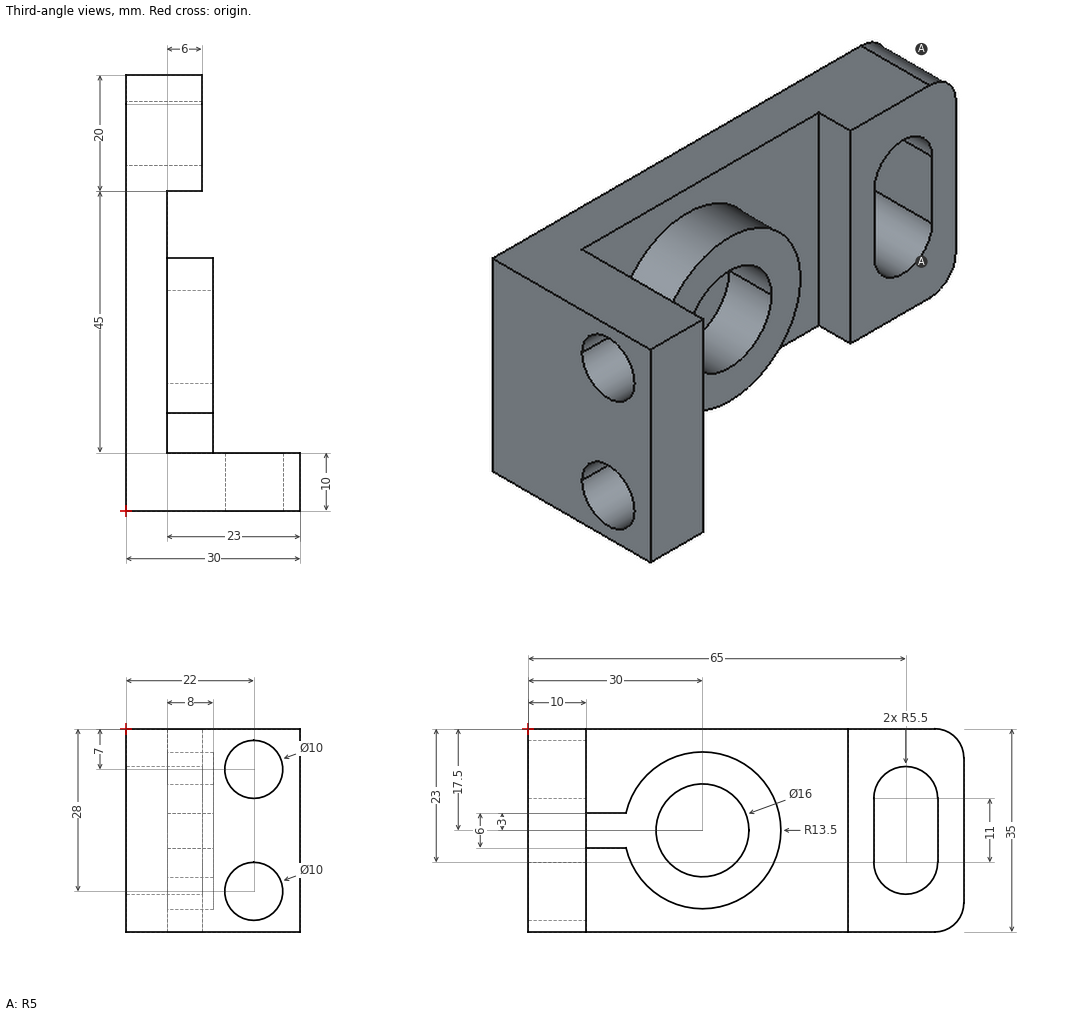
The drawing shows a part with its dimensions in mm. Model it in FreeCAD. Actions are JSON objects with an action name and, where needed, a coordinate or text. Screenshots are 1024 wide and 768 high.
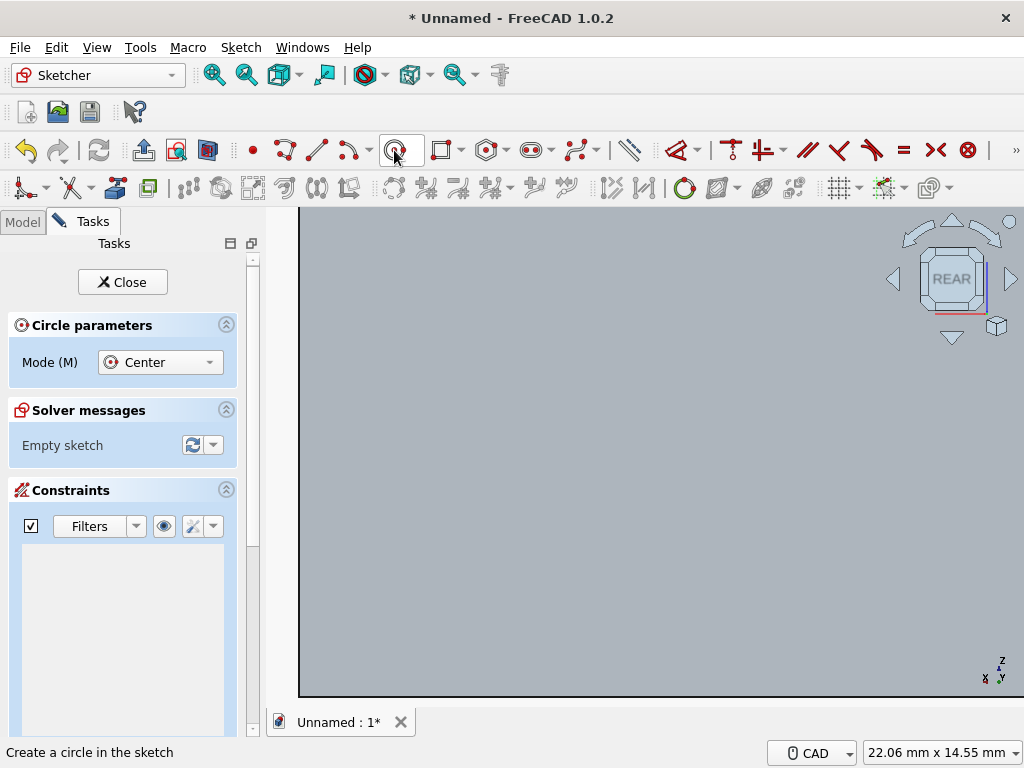
{"action": "left_click", "coordinate": [574, 456]}
{"action": "left_click", "coordinate": [695, 335]}
{"action": "key", "text": "Escape"}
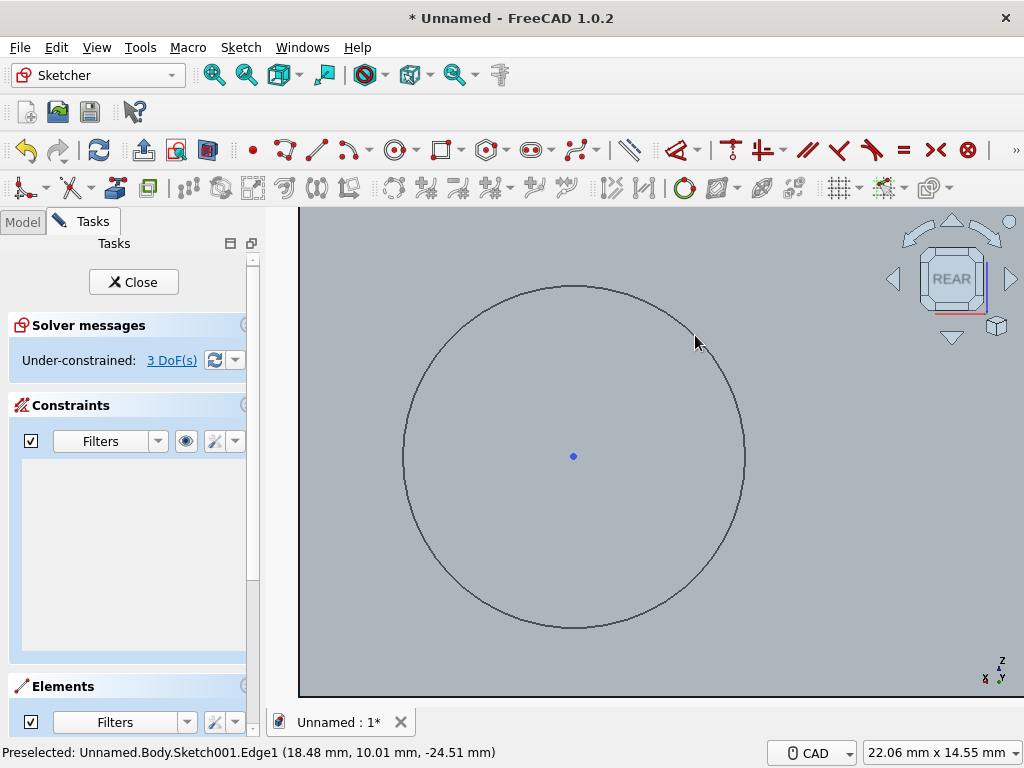
{"action": "left_click", "coordinate": [676, 150]}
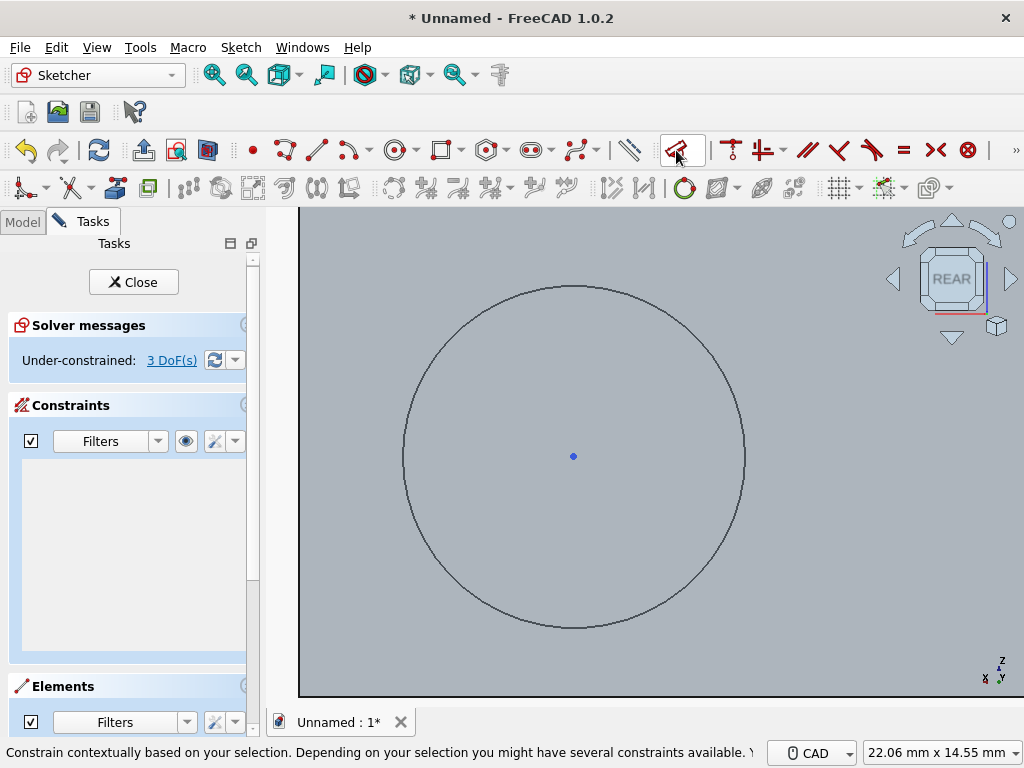
{"action": "left_click", "coordinate": [695, 336]}
{"action": "left_click", "coordinate": [718, 313]}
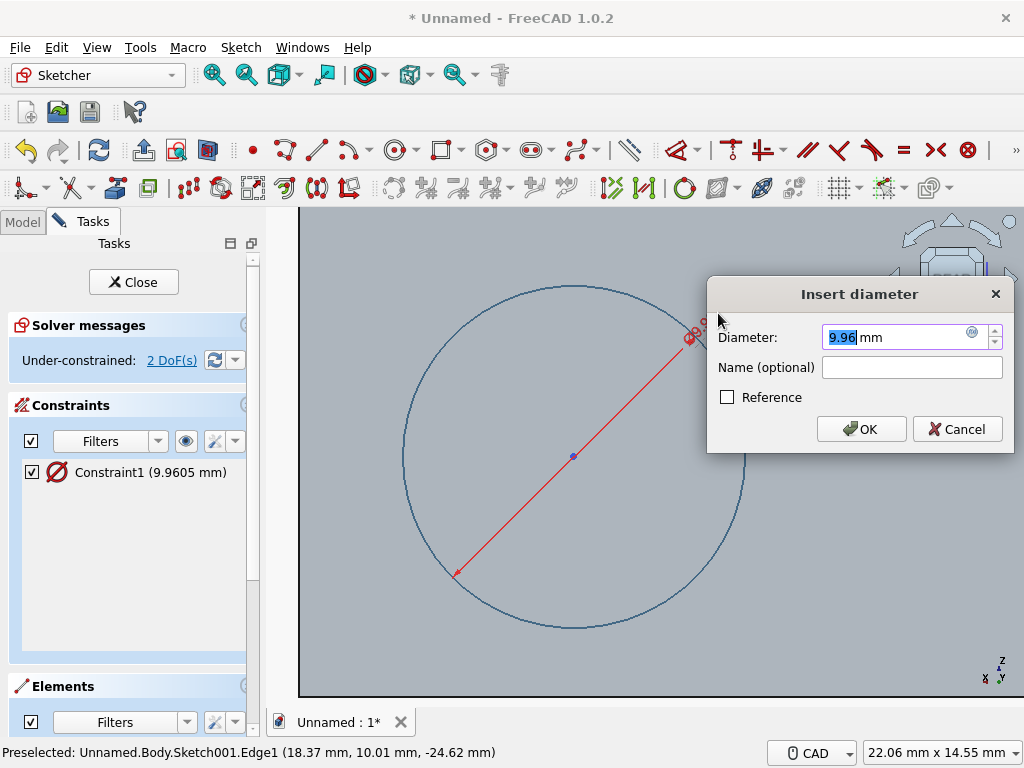
{"action": "type", "text": "10"}
{"action": "key", "text": "Return"}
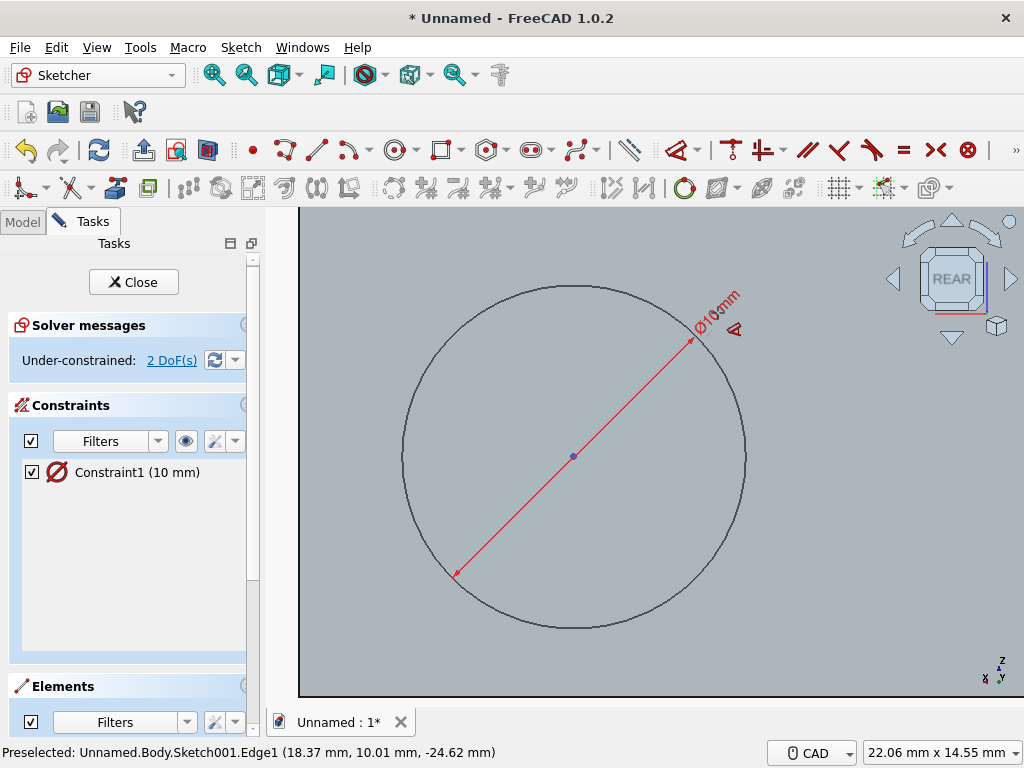
{"action": "left_click", "coordinate": [574, 457]}
{"action": "left_click", "coordinate": [716, 491]}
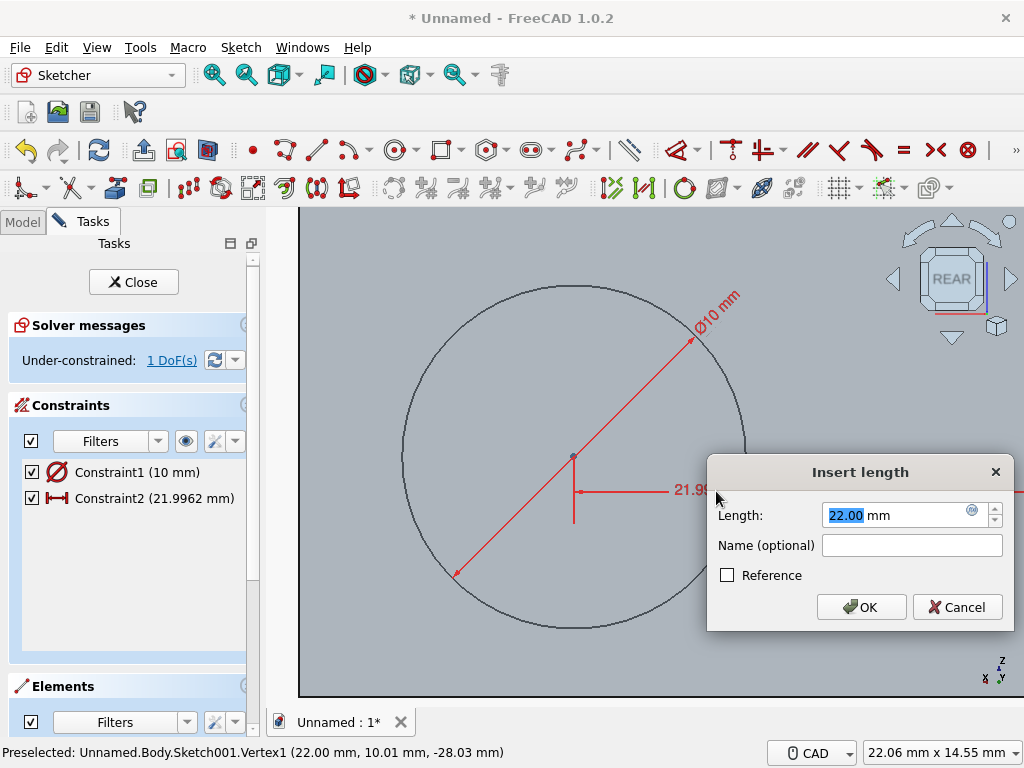
{"action": "type", "text": "22"}
{"action": "key", "text": "Return"}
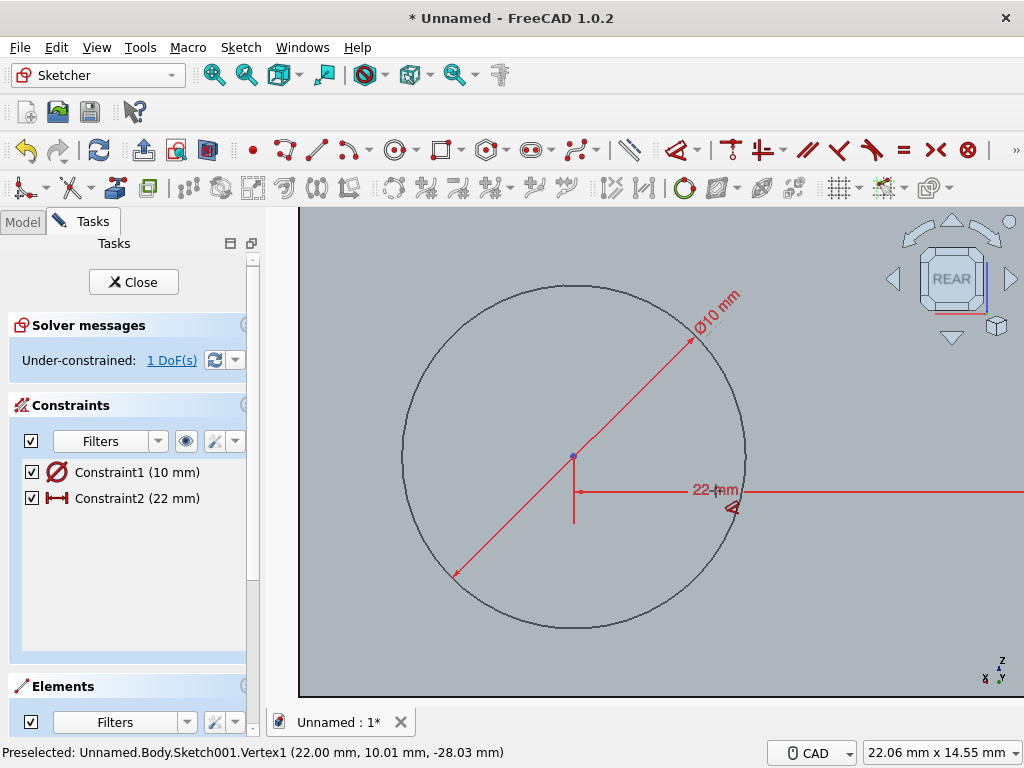
{"action": "left_click", "coordinate": [574, 457]}
{"action": "left_click", "coordinate": [540, 346]}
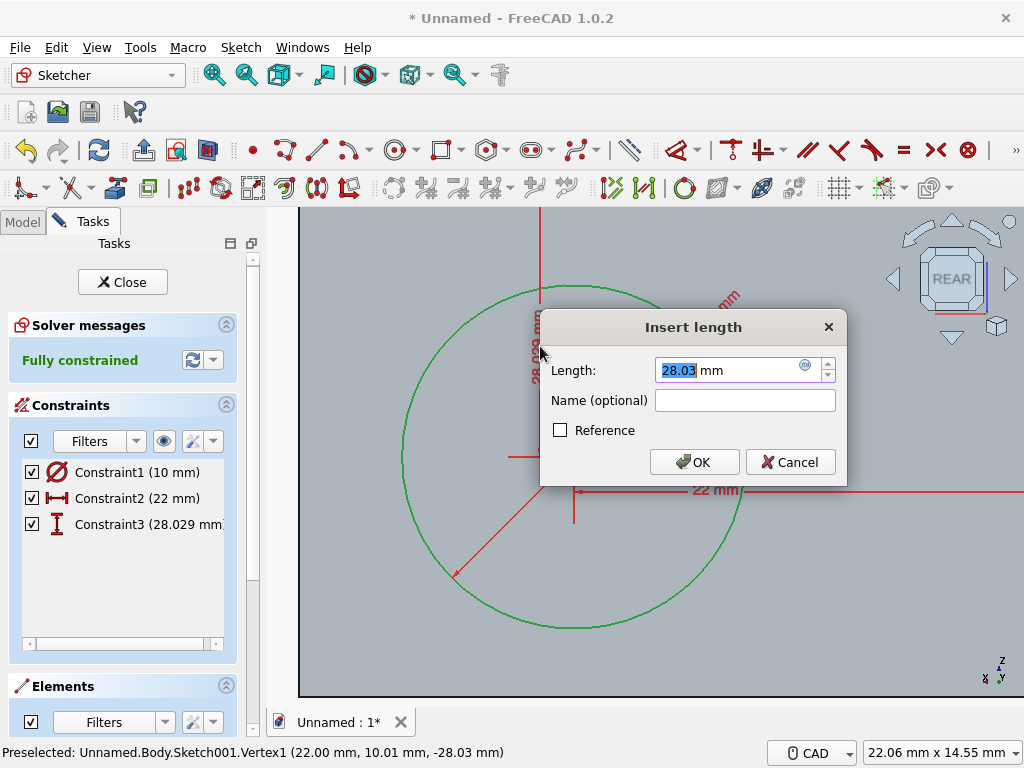
{"action": "type", "text": "28"}
{"action": "key", "text": "Return"}
{"action": "key", "text": "Escape"}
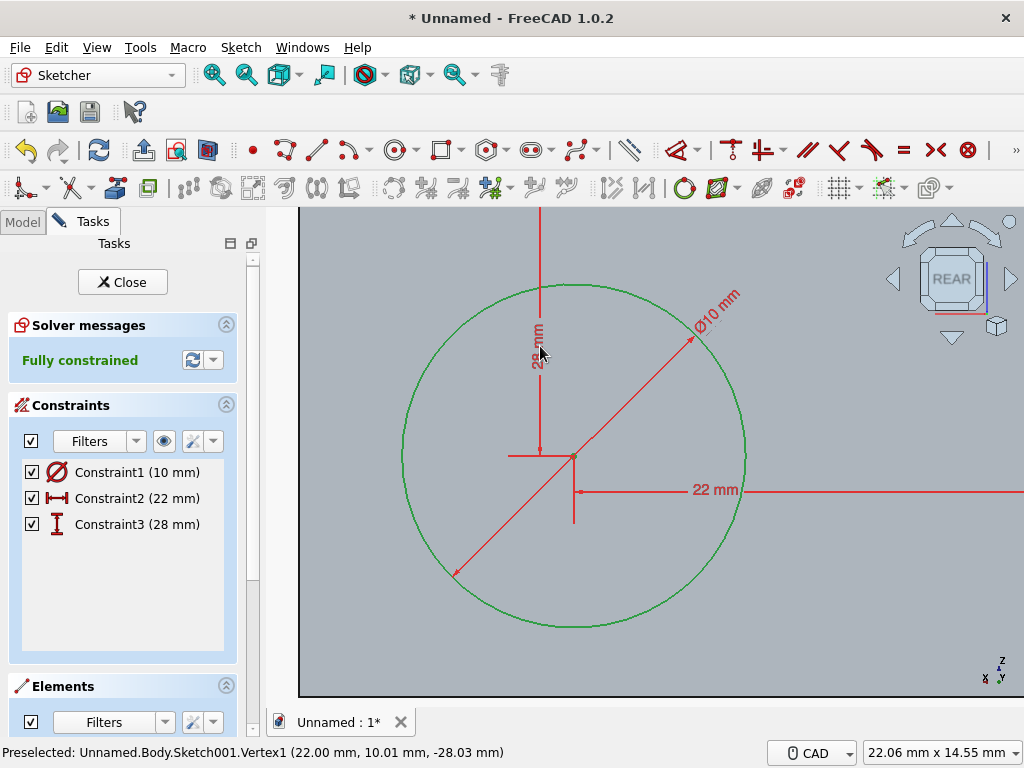
{"action": "left_click", "coordinate": [123, 282]}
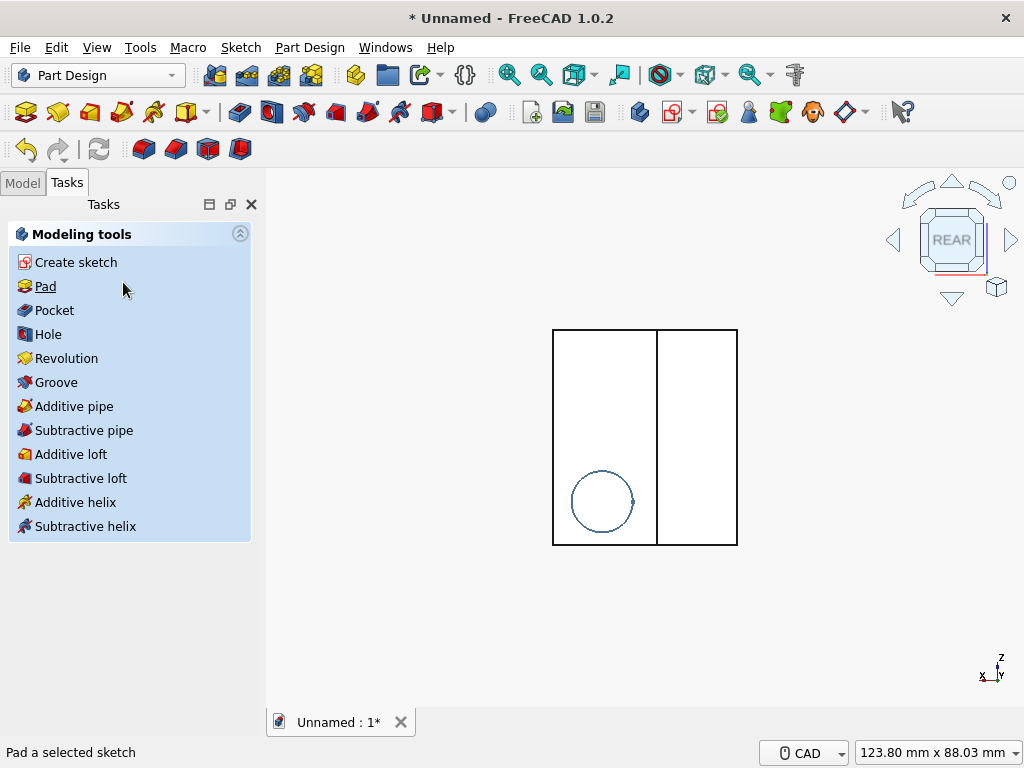
{"action": "left_click", "coordinate": [240, 112]}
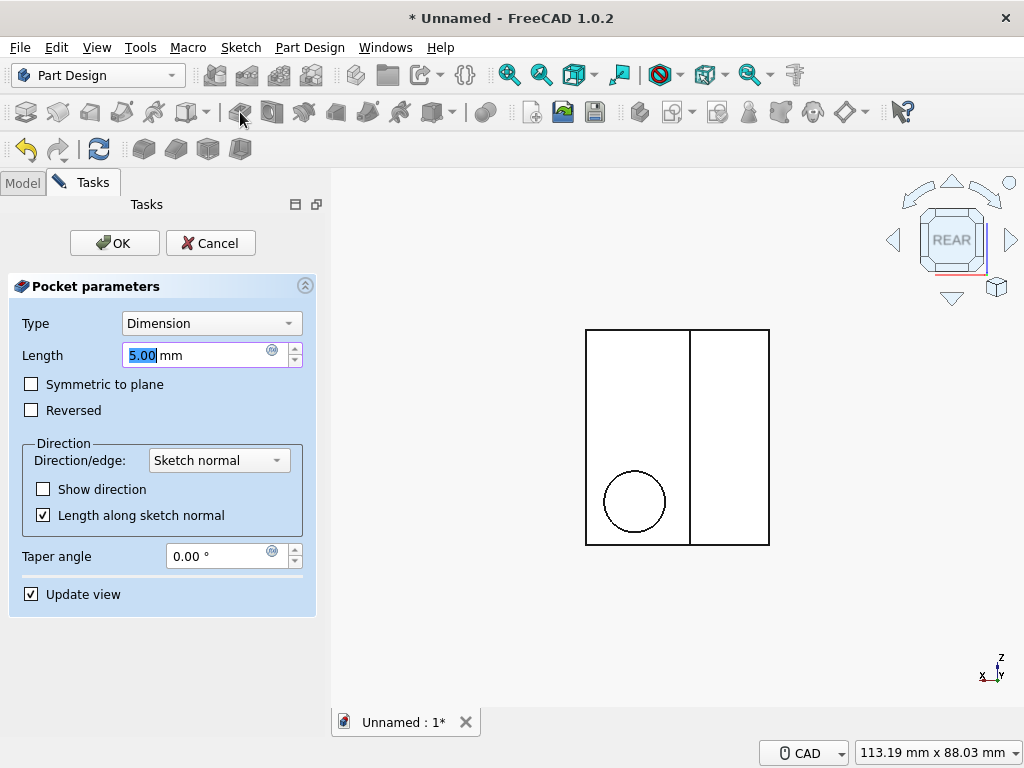
{"action": "left_click", "coordinate": [212, 324]}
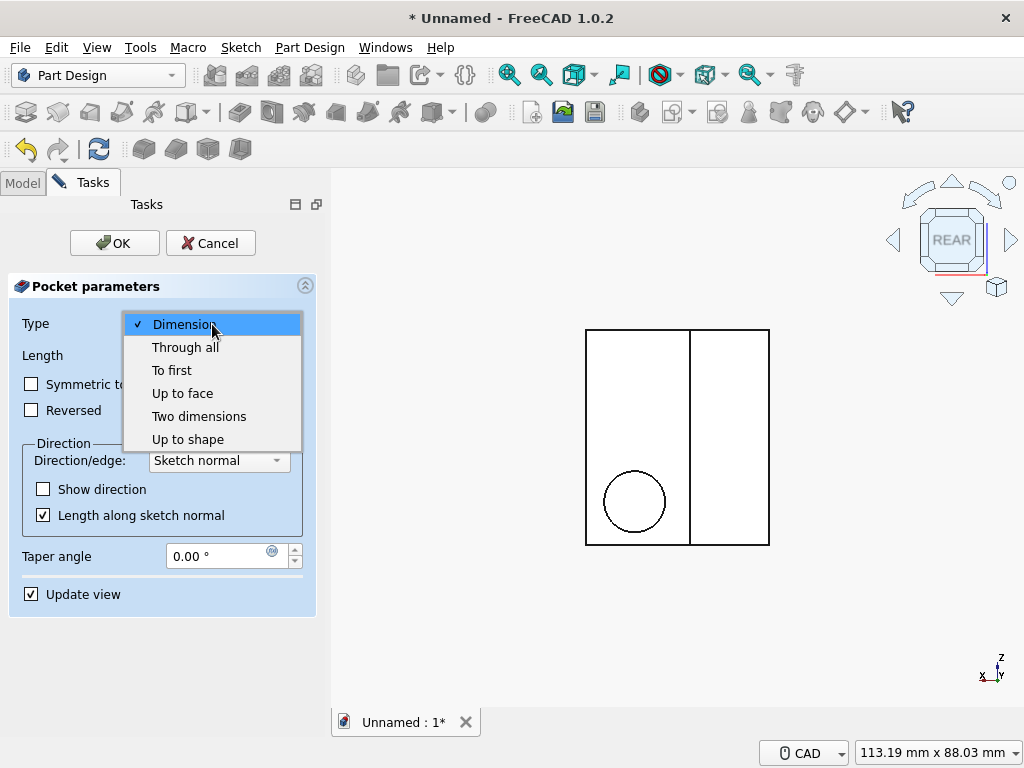
{"action": "left_click", "coordinate": [212, 370]}